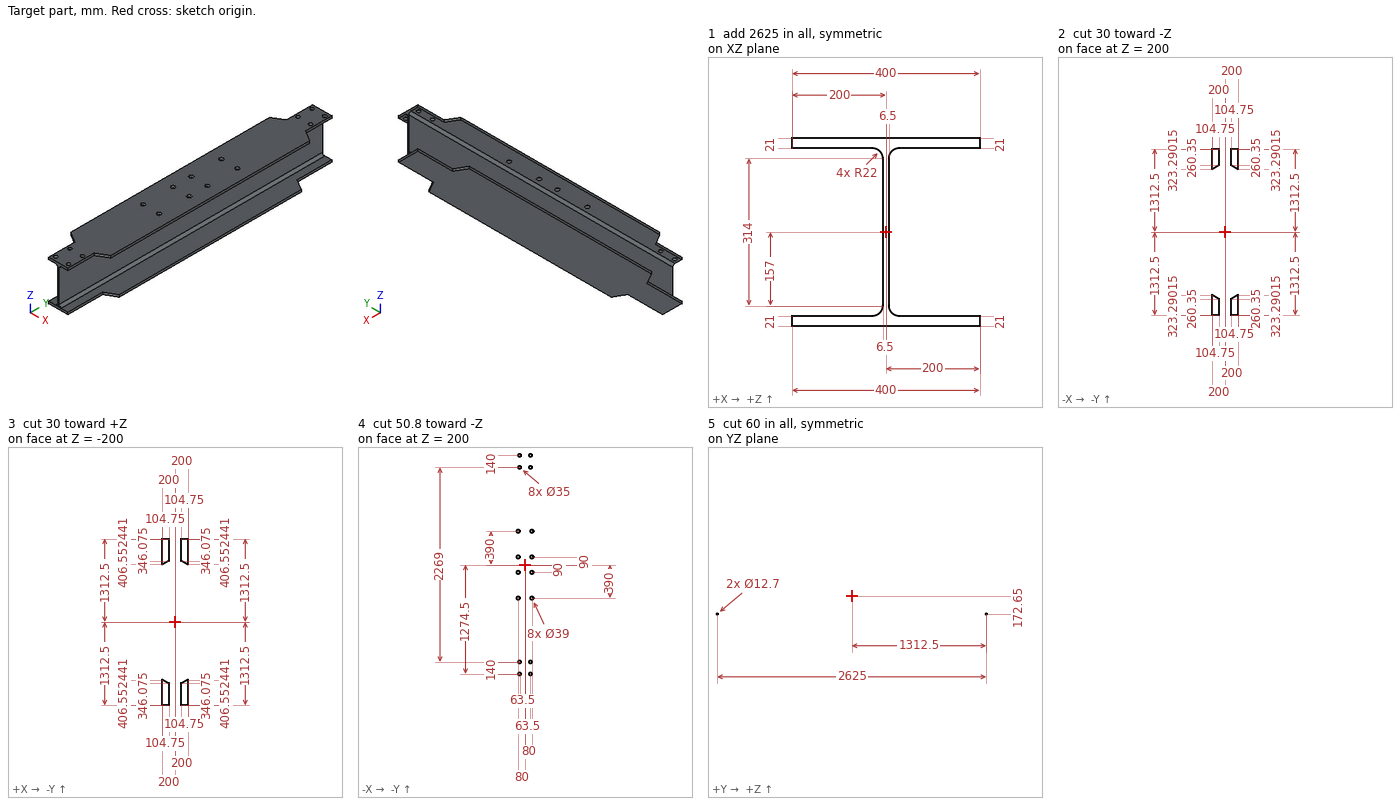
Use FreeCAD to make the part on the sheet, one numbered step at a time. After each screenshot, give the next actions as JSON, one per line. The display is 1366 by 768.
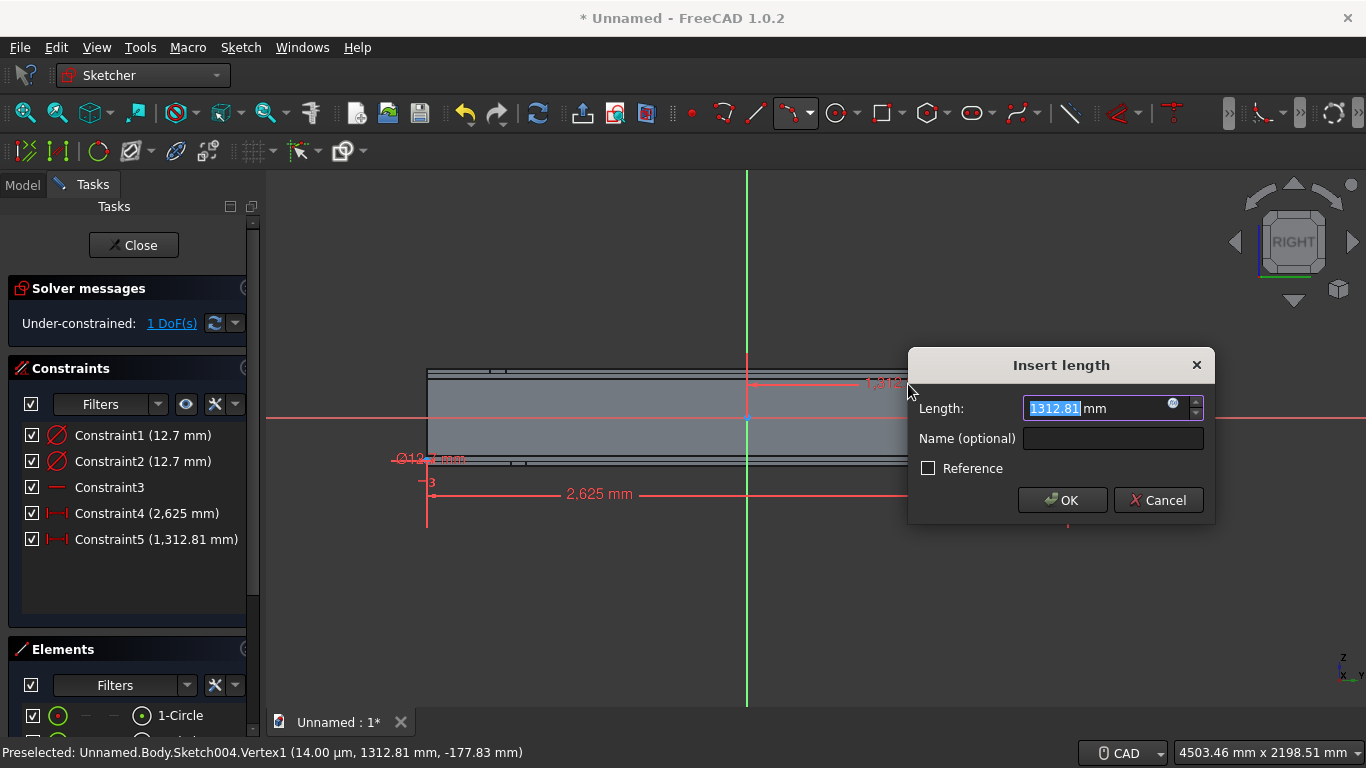
{"action": "type", "text": "1312.5"}
{"action": "key", "text": "Return"}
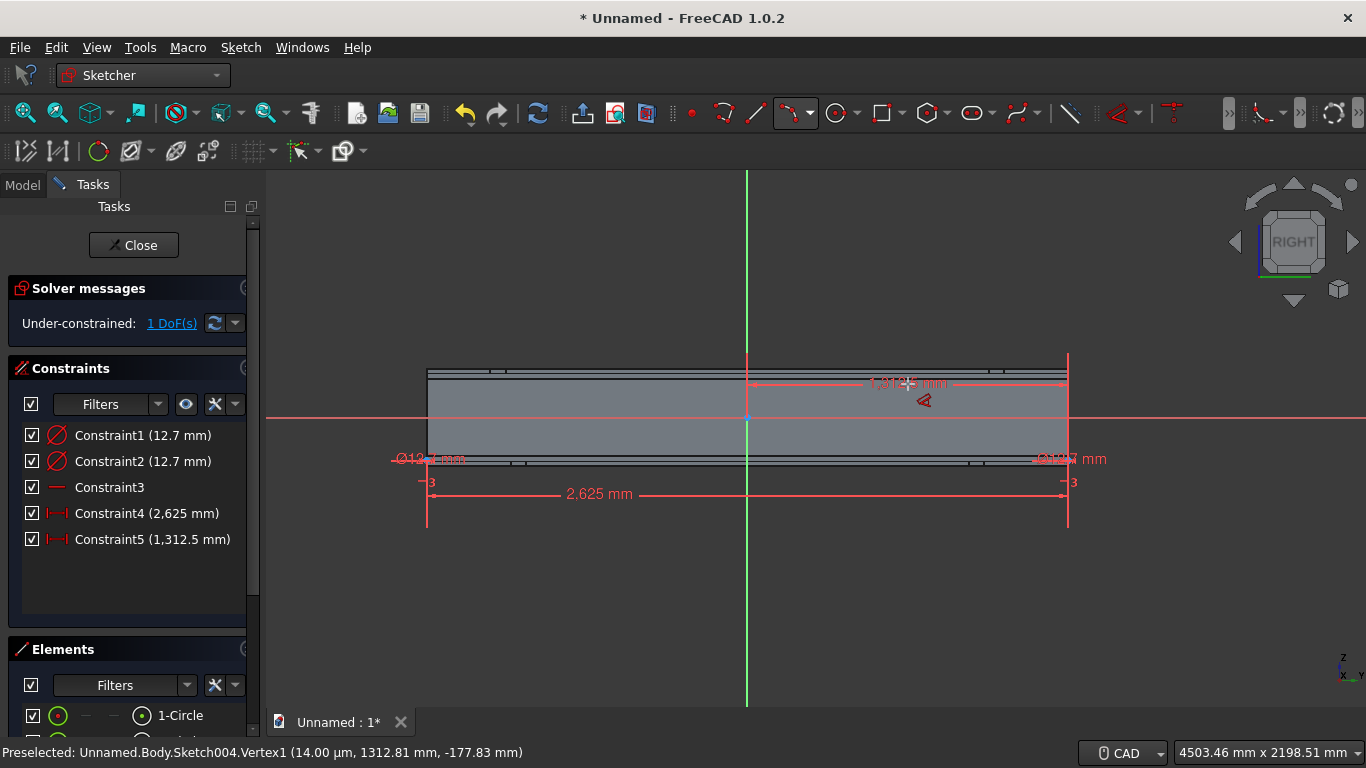
{"action": "left_click", "coordinate": [1068, 461]}
{"action": "left_click", "coordinate": [1102, 439]}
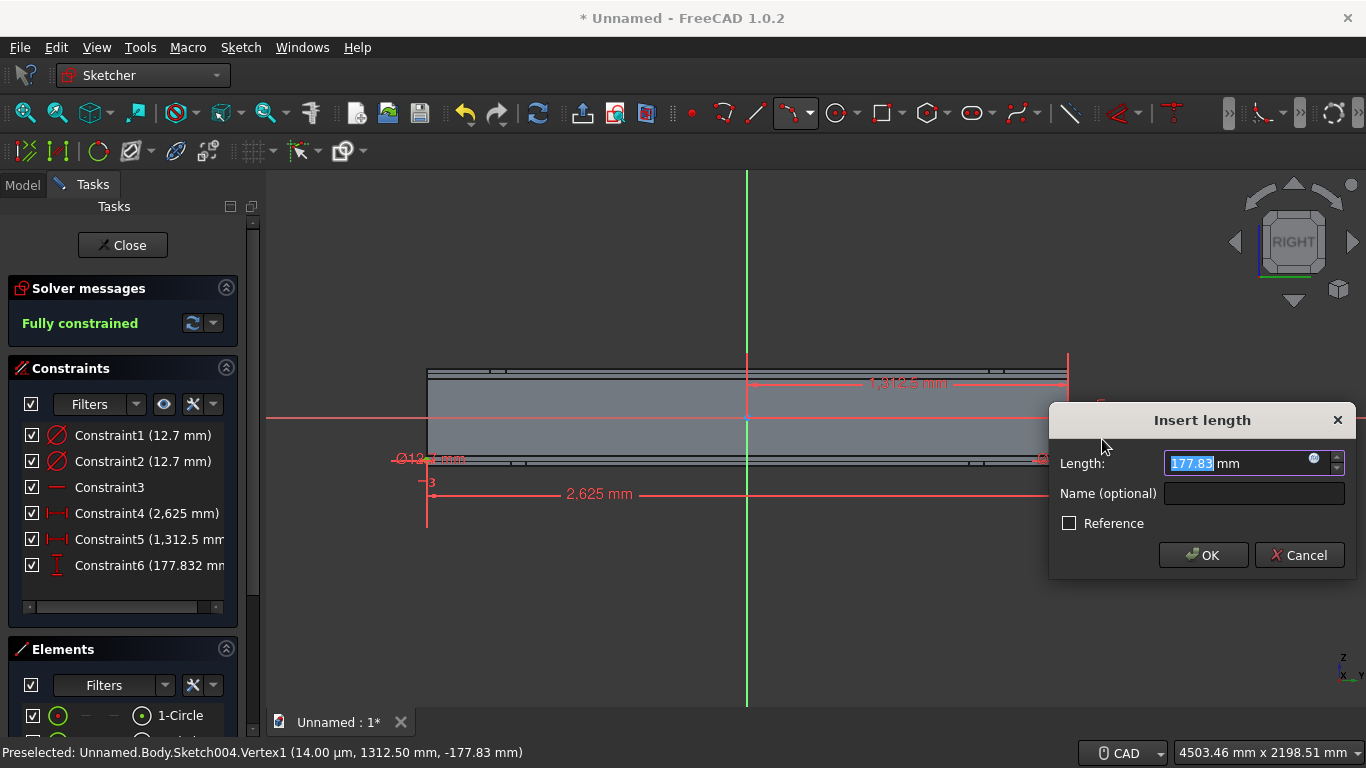
{"action": "type", "text": "172.65"}
{"action": "key", "text": "Return"}
{"action": "key", "text": "Escape"}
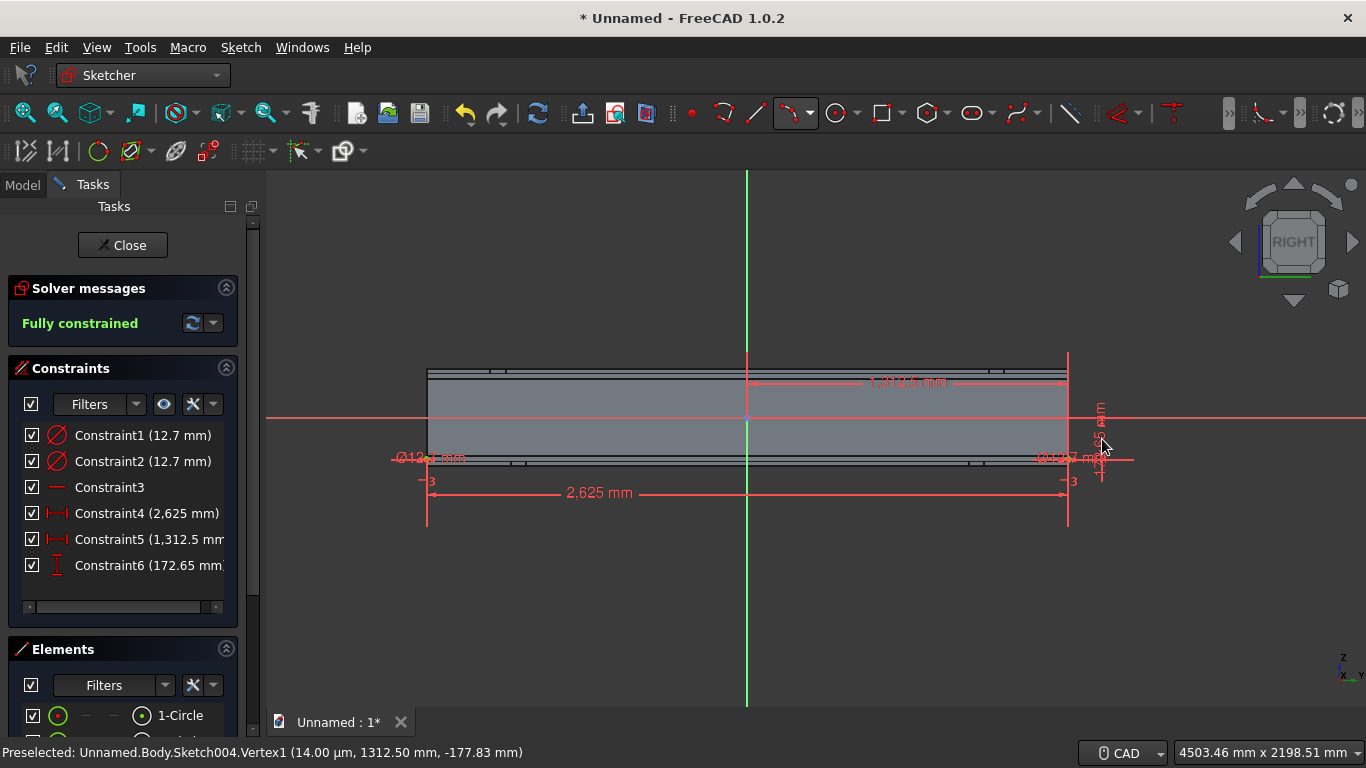
{"action": "left_click", "coordinate": [123, 245]}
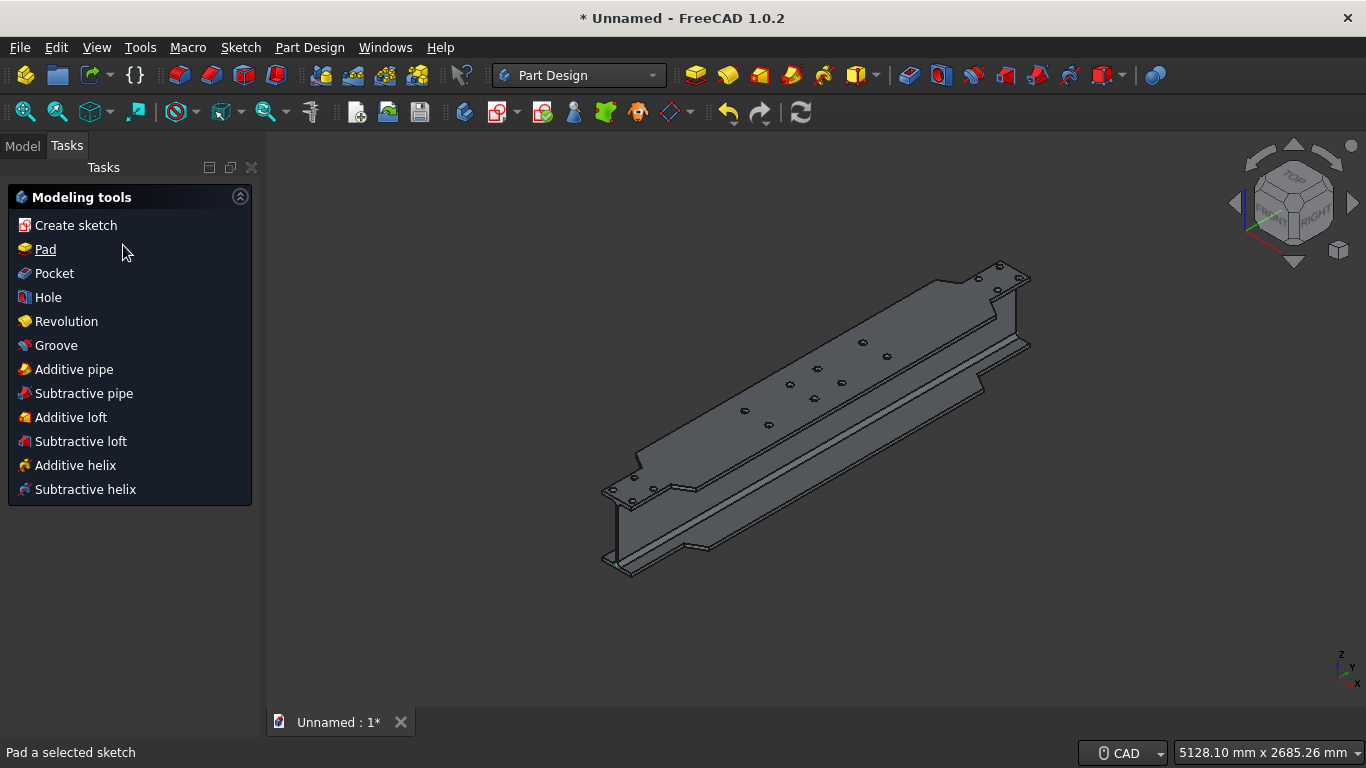
{"action": "left_click", "coordinate": [910, 76]}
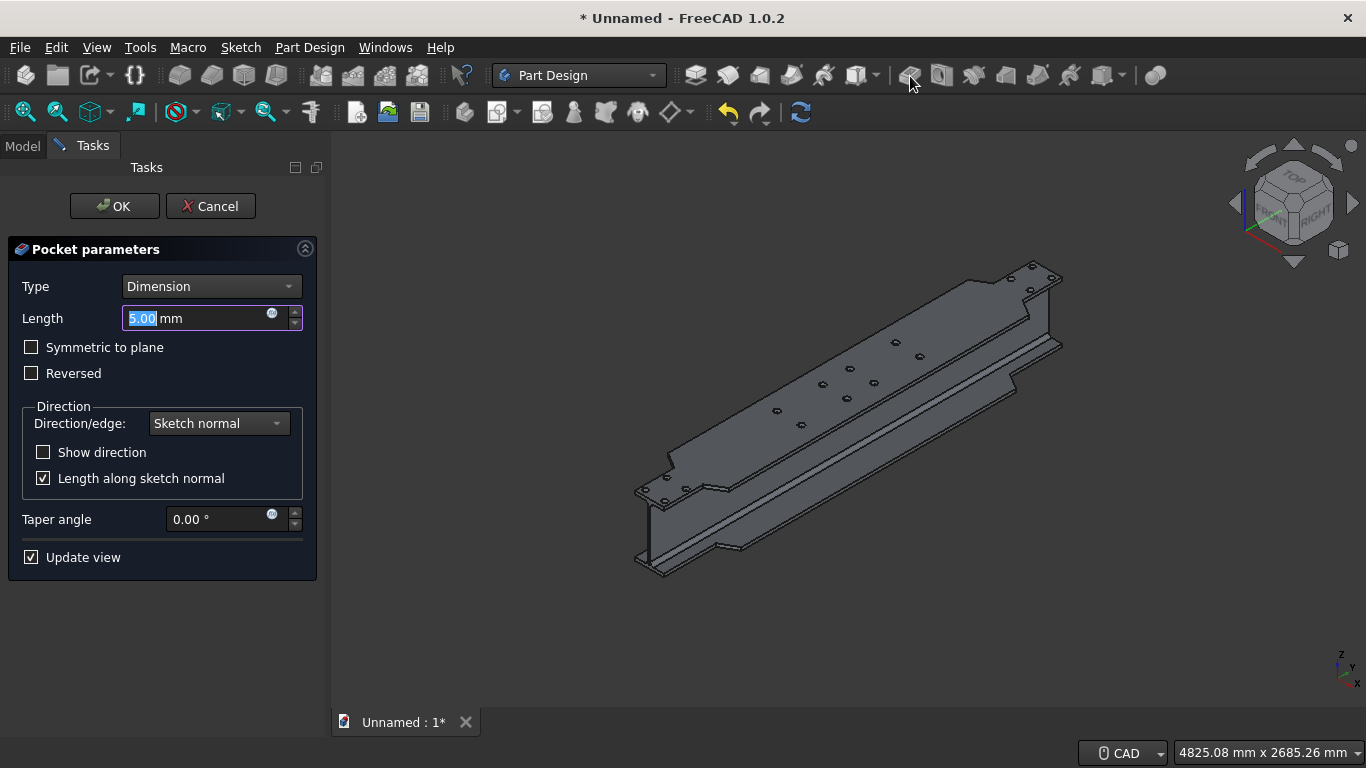
{"action": "type", "text": "60"}
{"action": "key", "text": "Tab"}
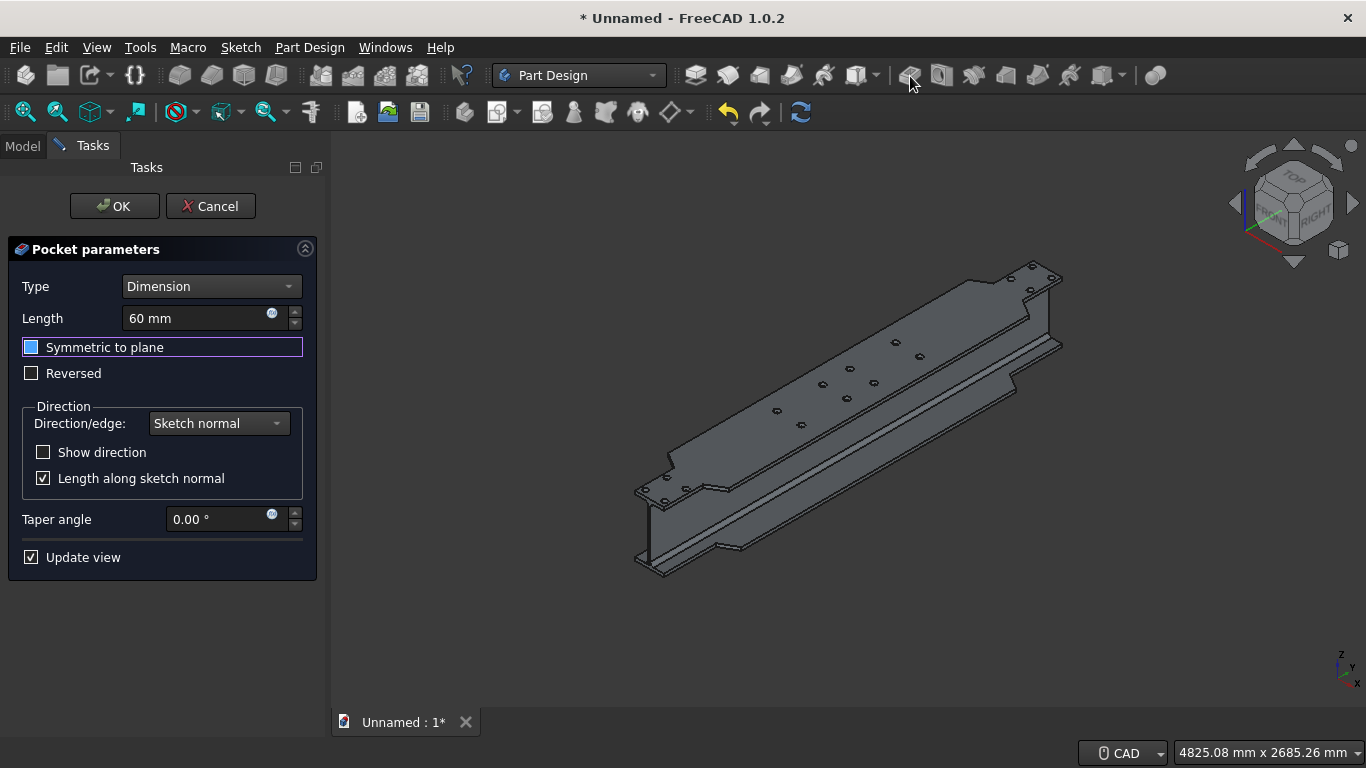
{"action": "left_click", "coordinate": [30, 347]}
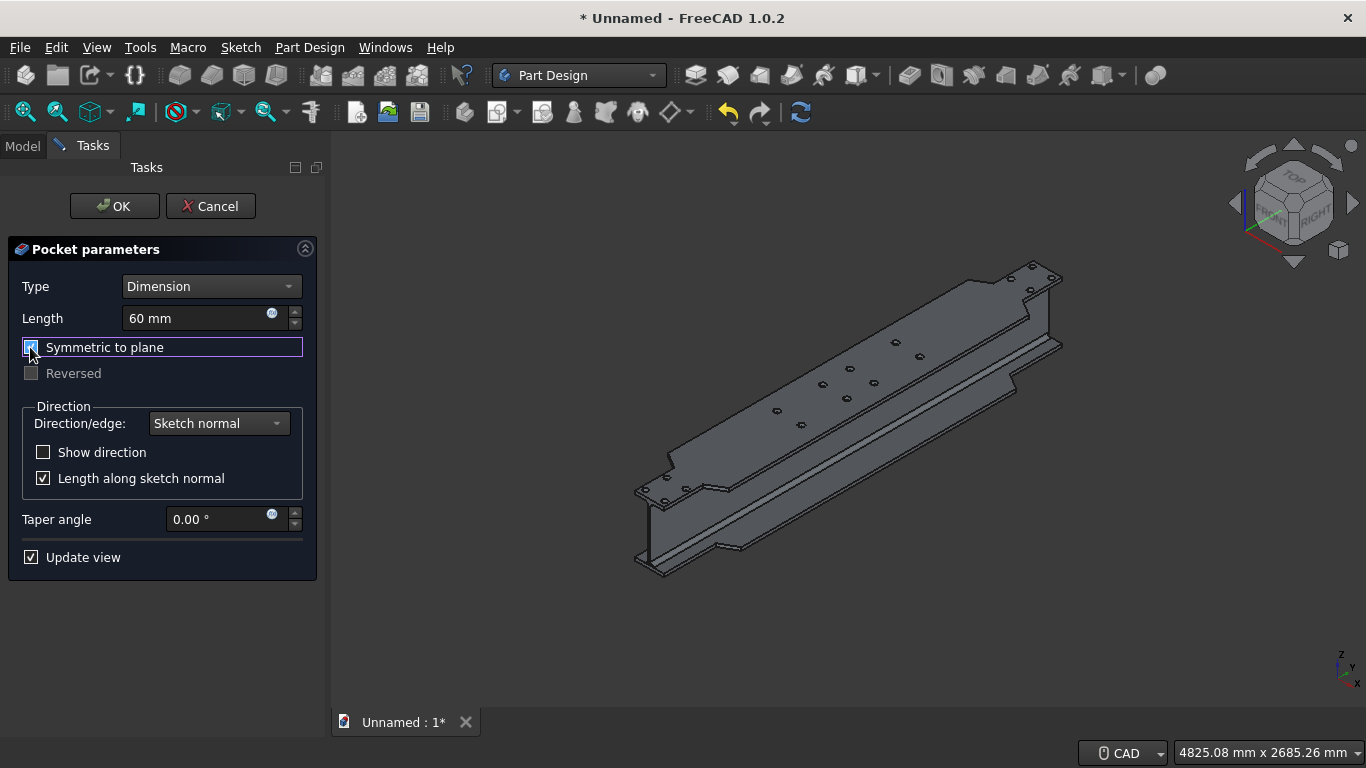
{"action": "left_click", "coordinate": [115, 206]}